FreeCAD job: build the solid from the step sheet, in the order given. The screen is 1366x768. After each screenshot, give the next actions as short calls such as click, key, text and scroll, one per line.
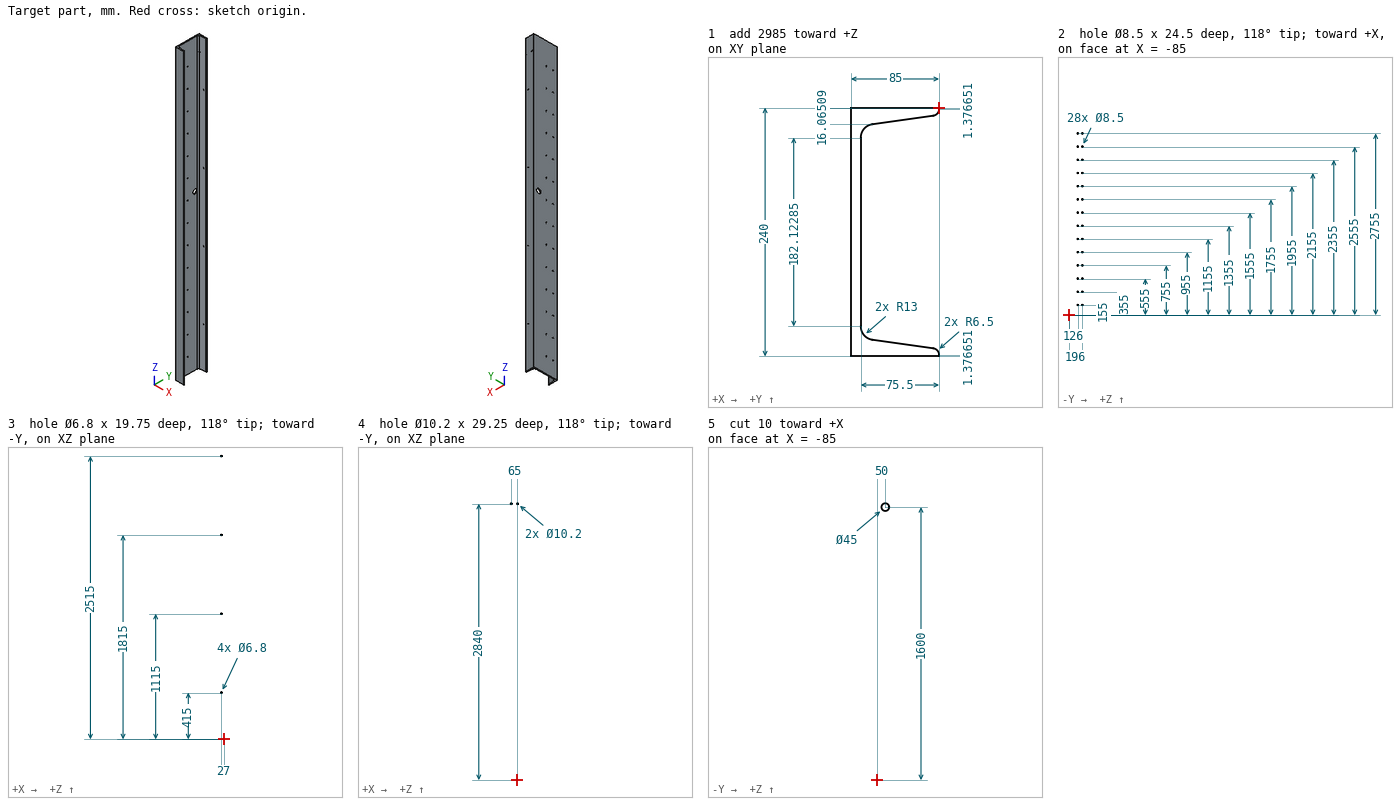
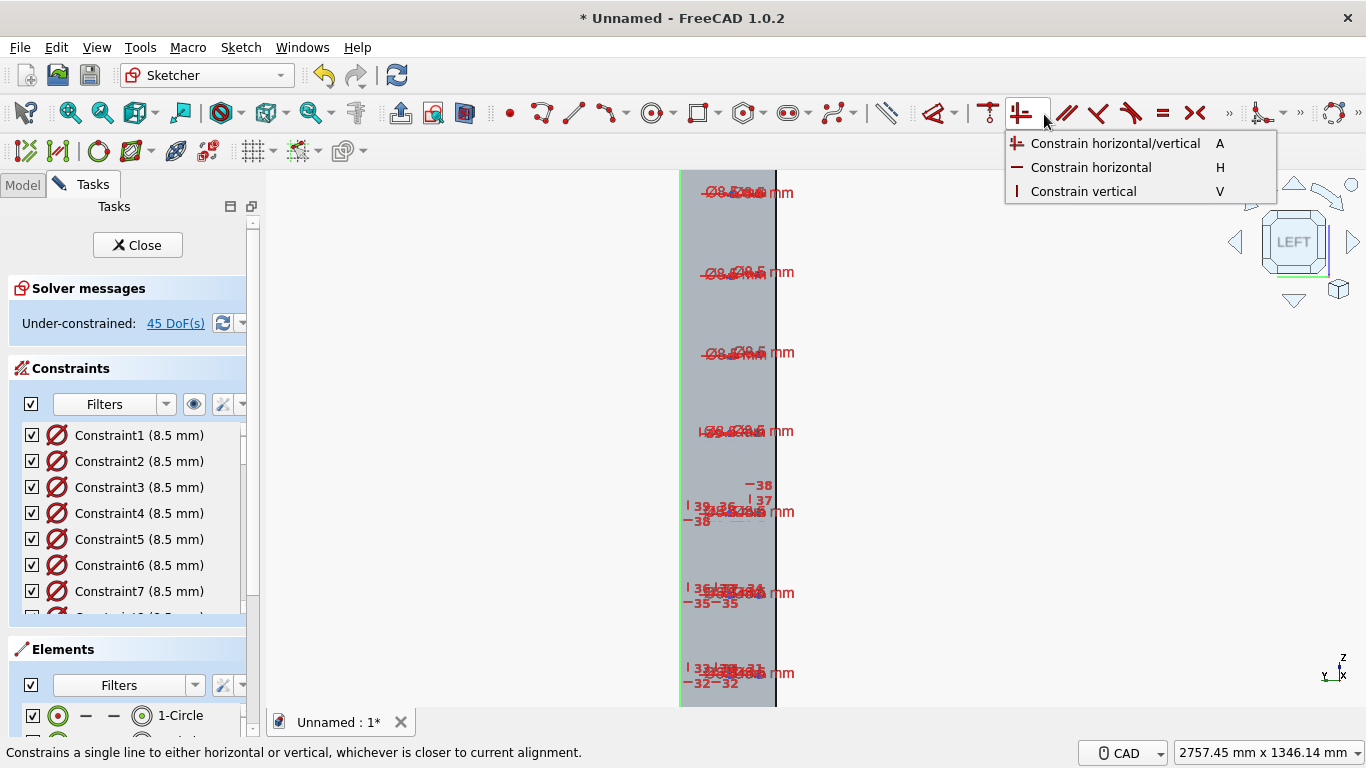
click(1141, 191)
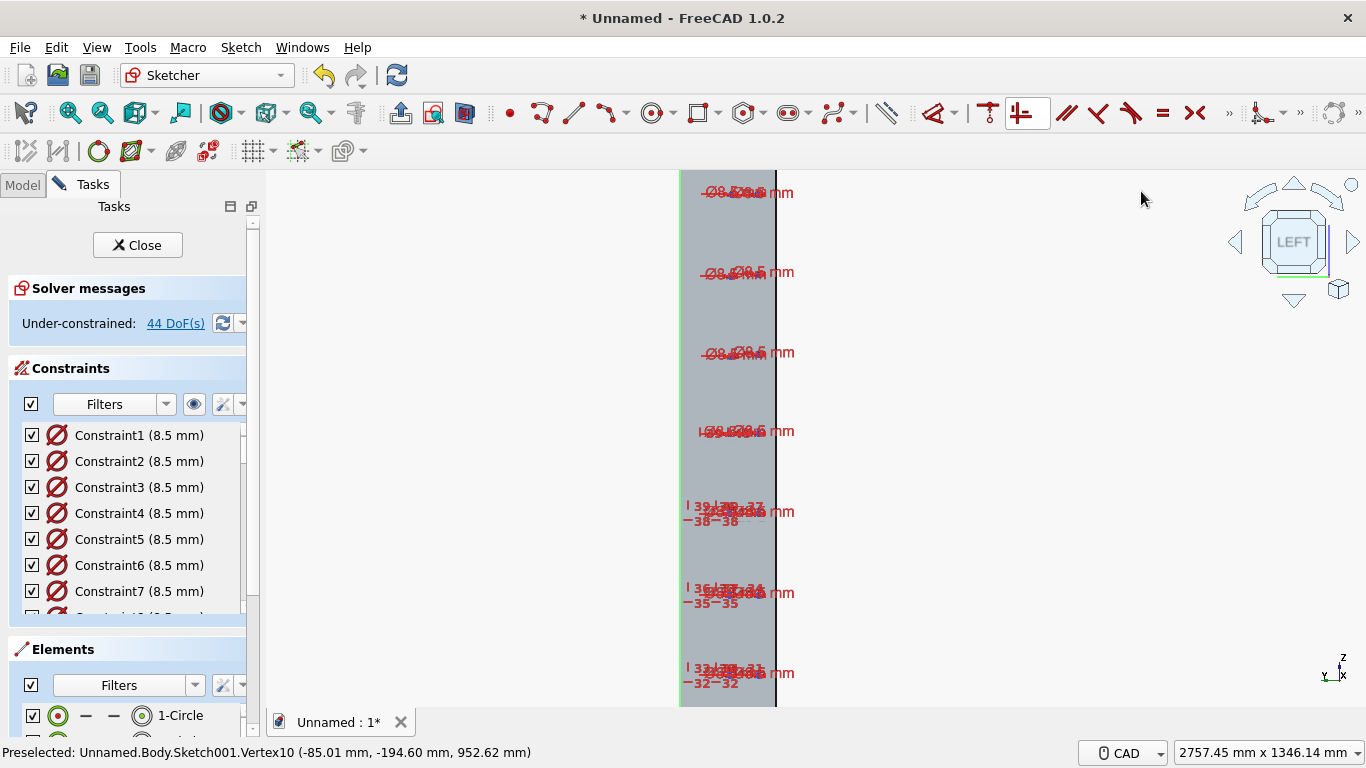
scroll(729, 434, up, 4)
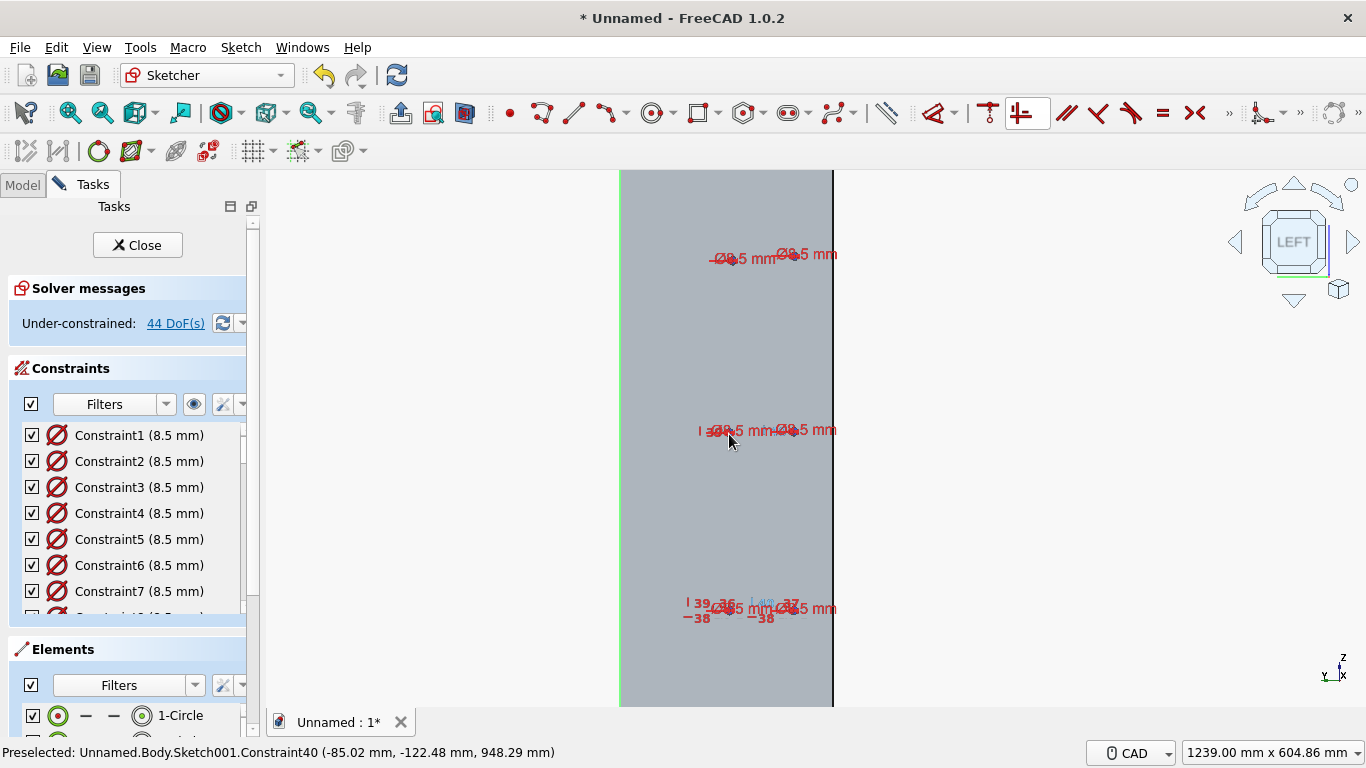
click(730, 433)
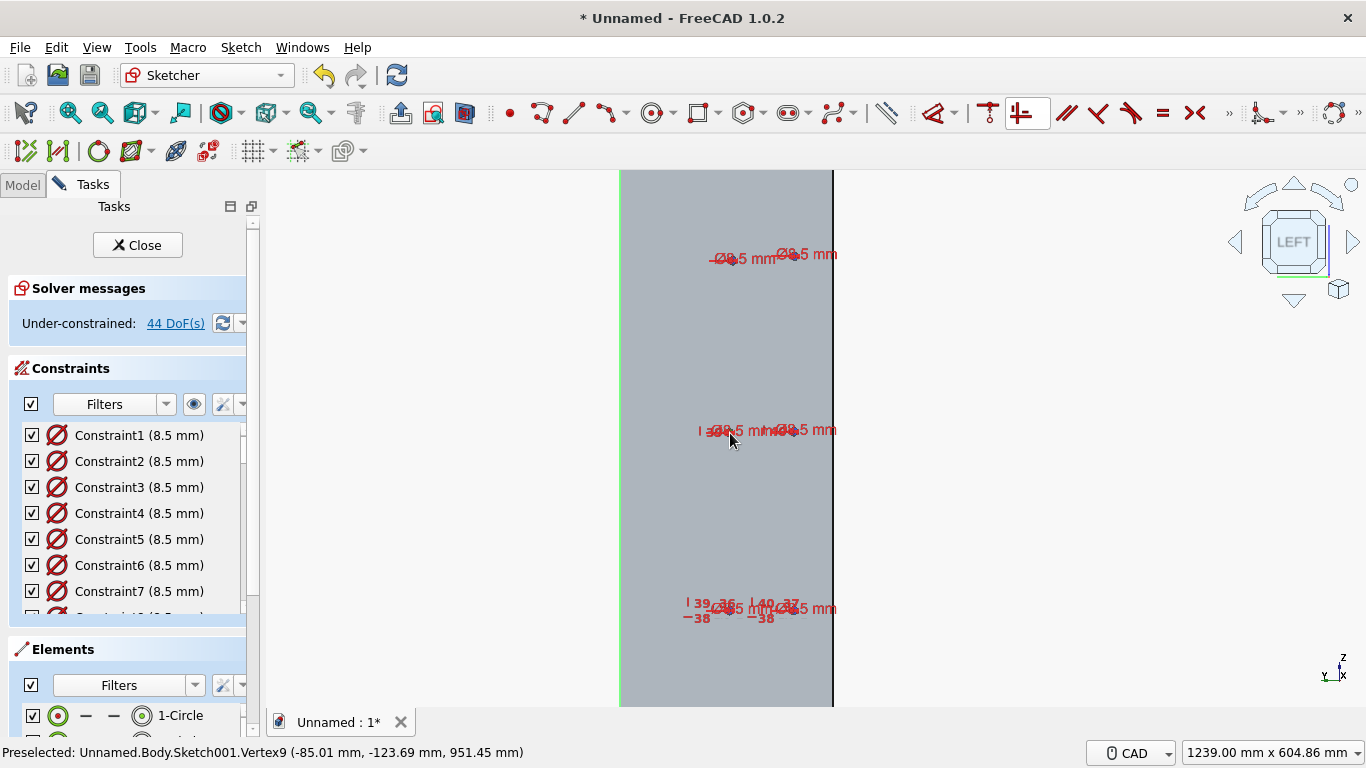
scroll(754, 499, down, 10)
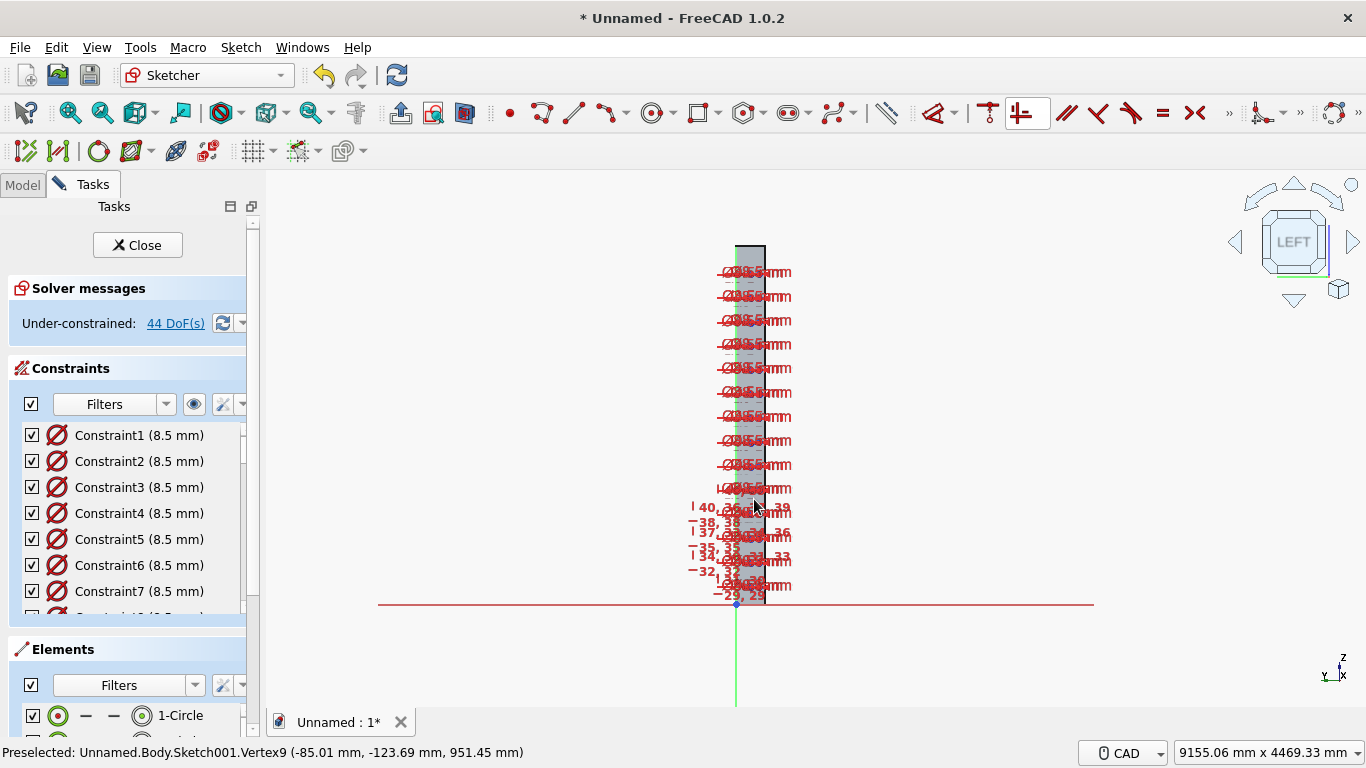
scroll(760, 490, up, 2)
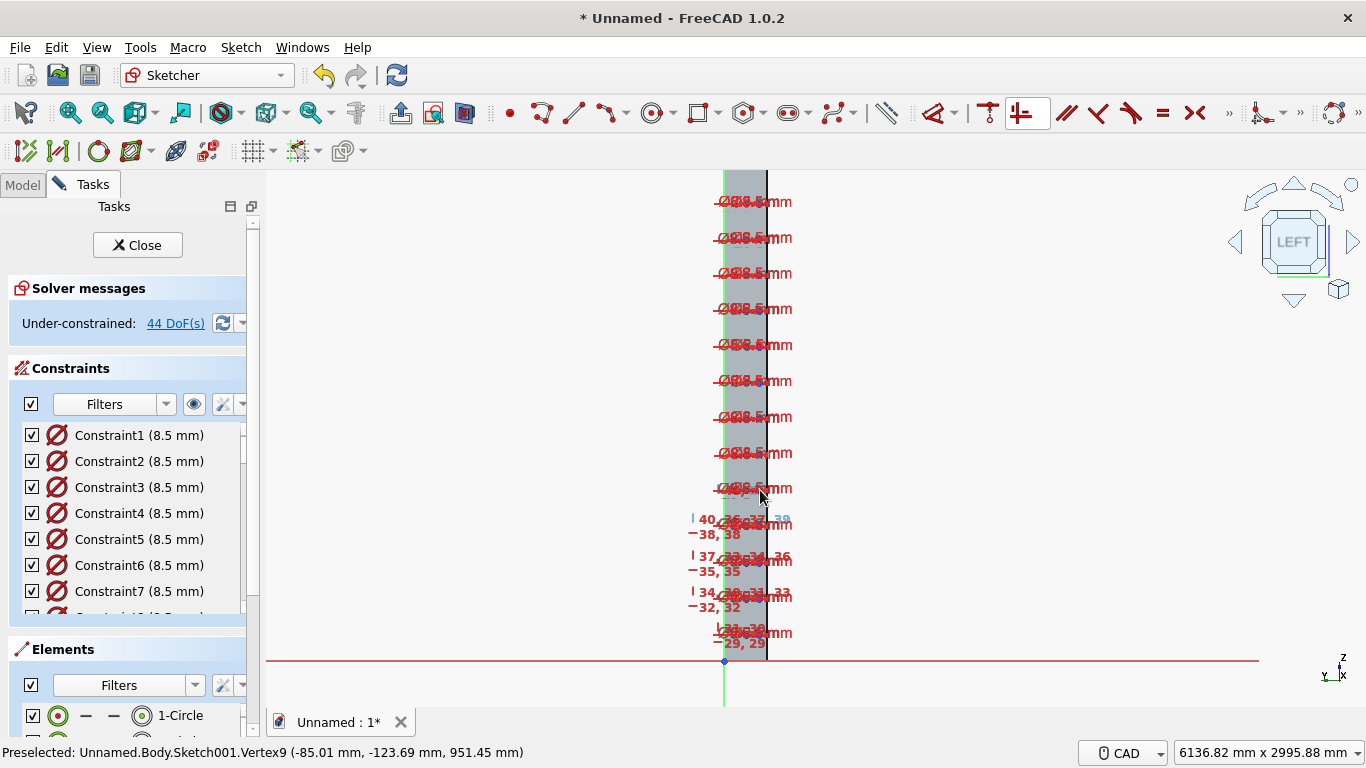
scroll(759, 490, up, 4)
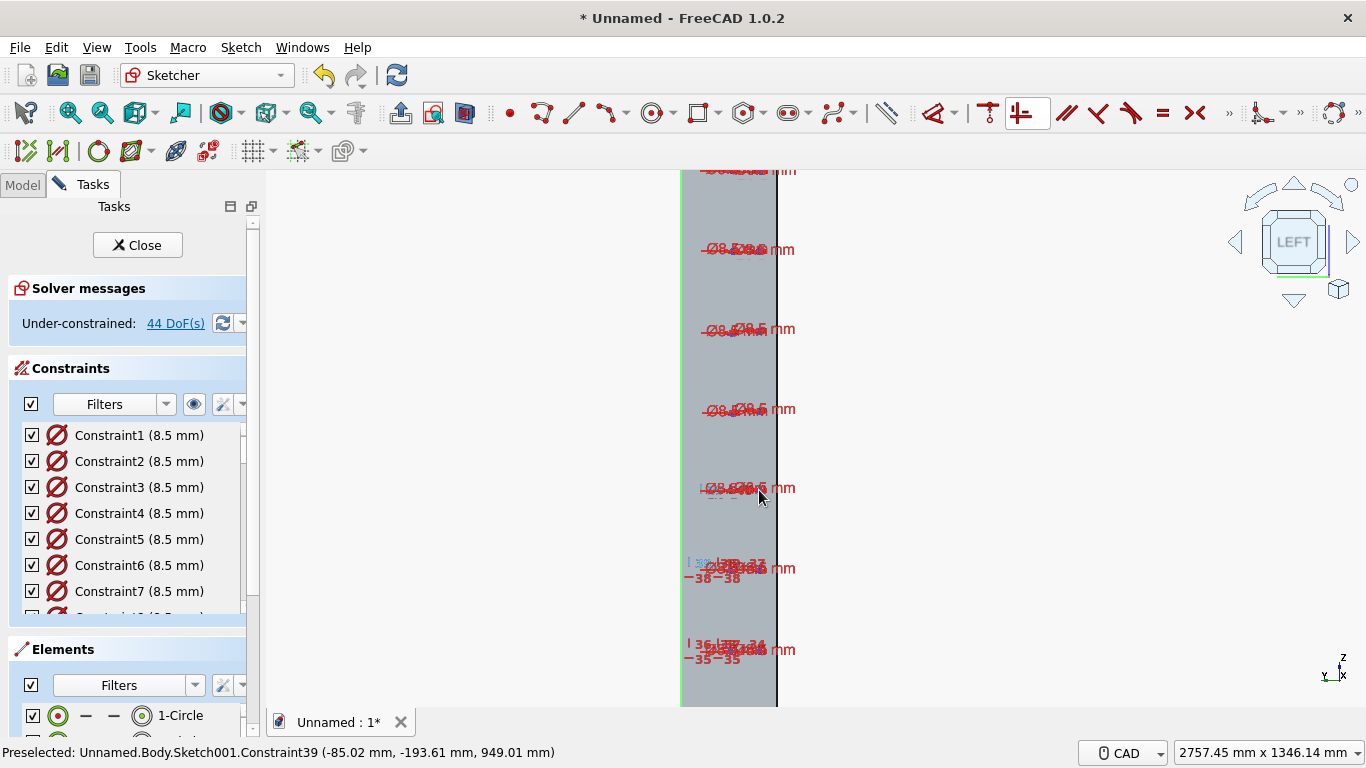
click(760, 490)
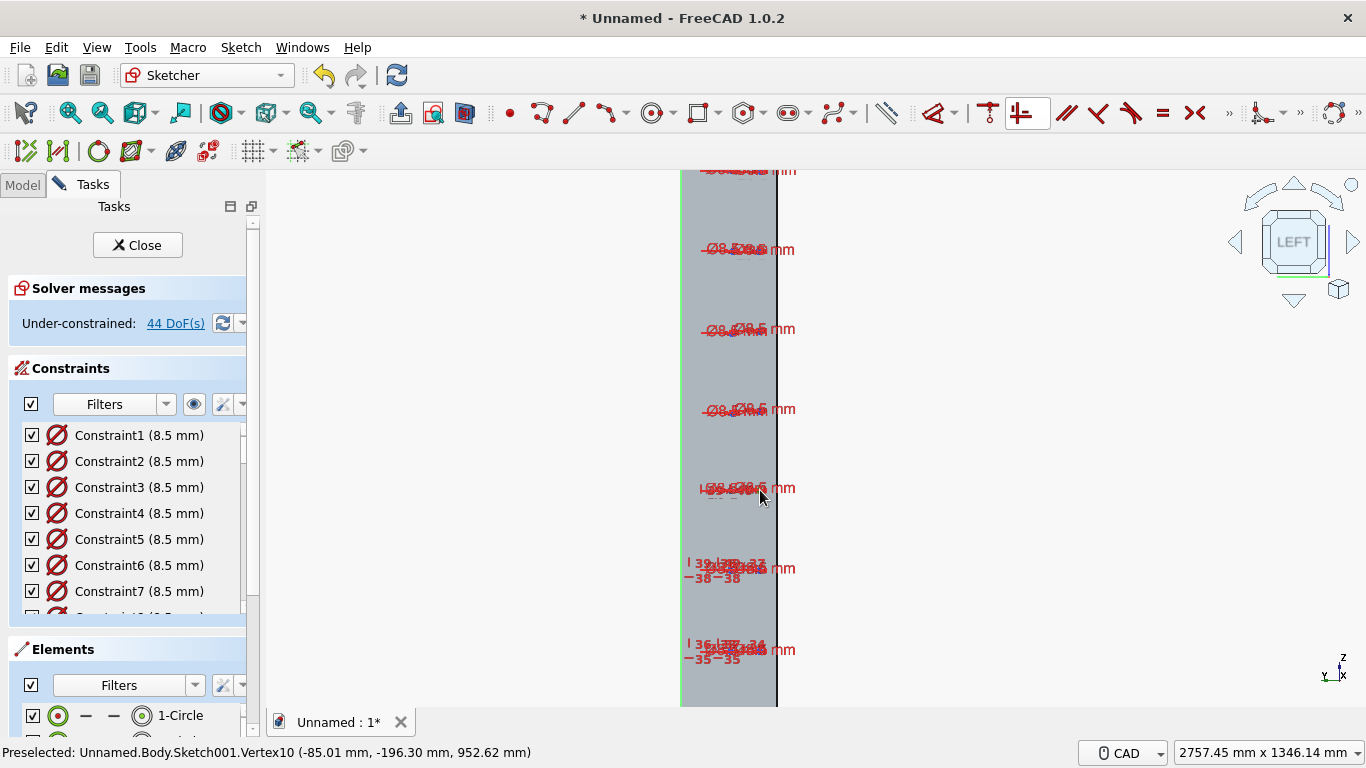
click(1044, 114)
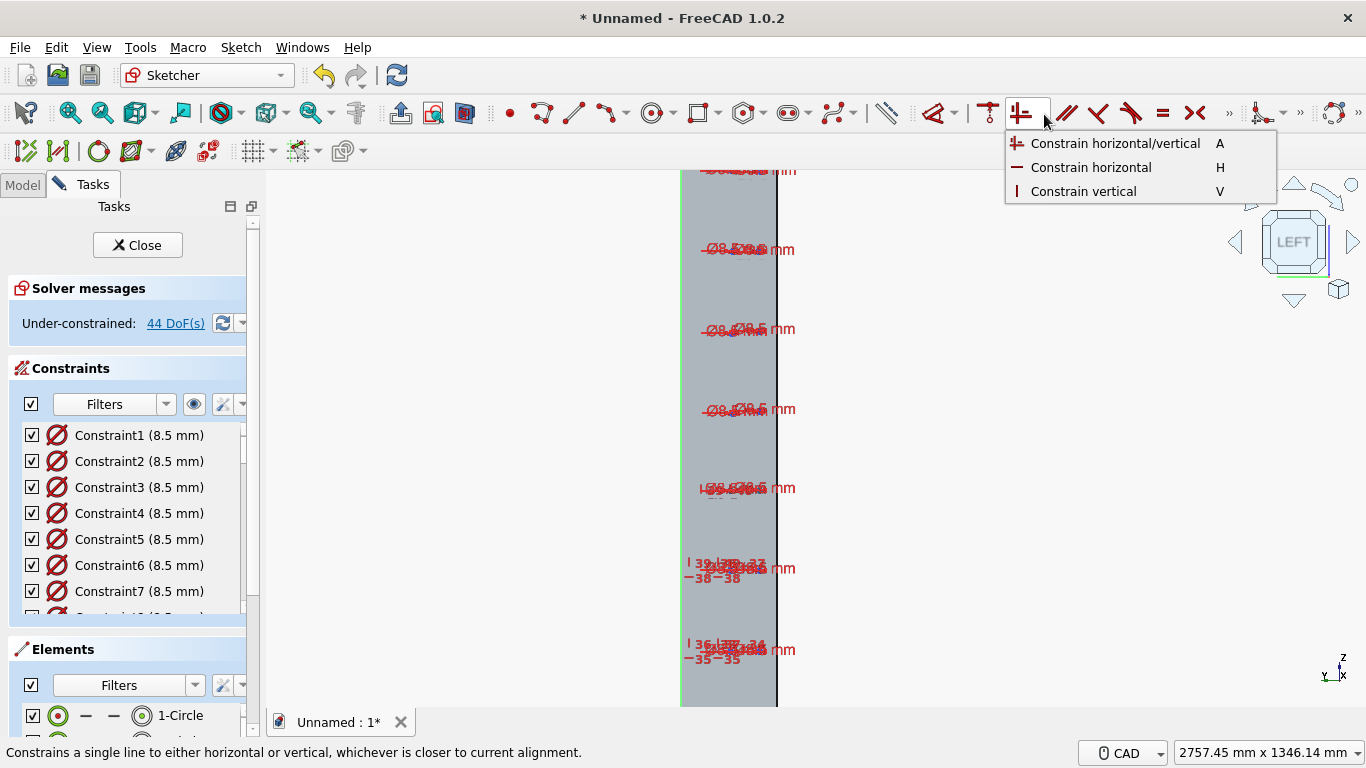
click(1141, 167)